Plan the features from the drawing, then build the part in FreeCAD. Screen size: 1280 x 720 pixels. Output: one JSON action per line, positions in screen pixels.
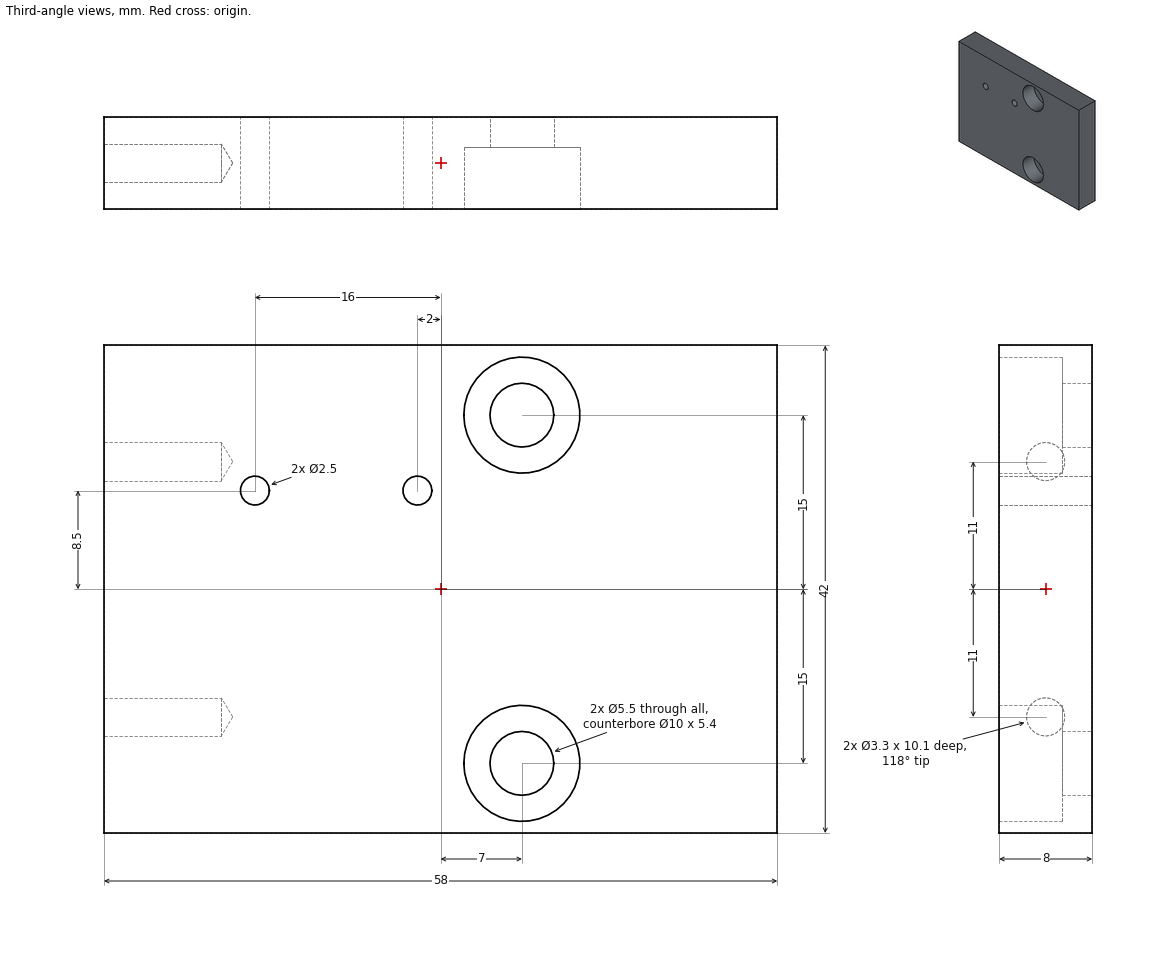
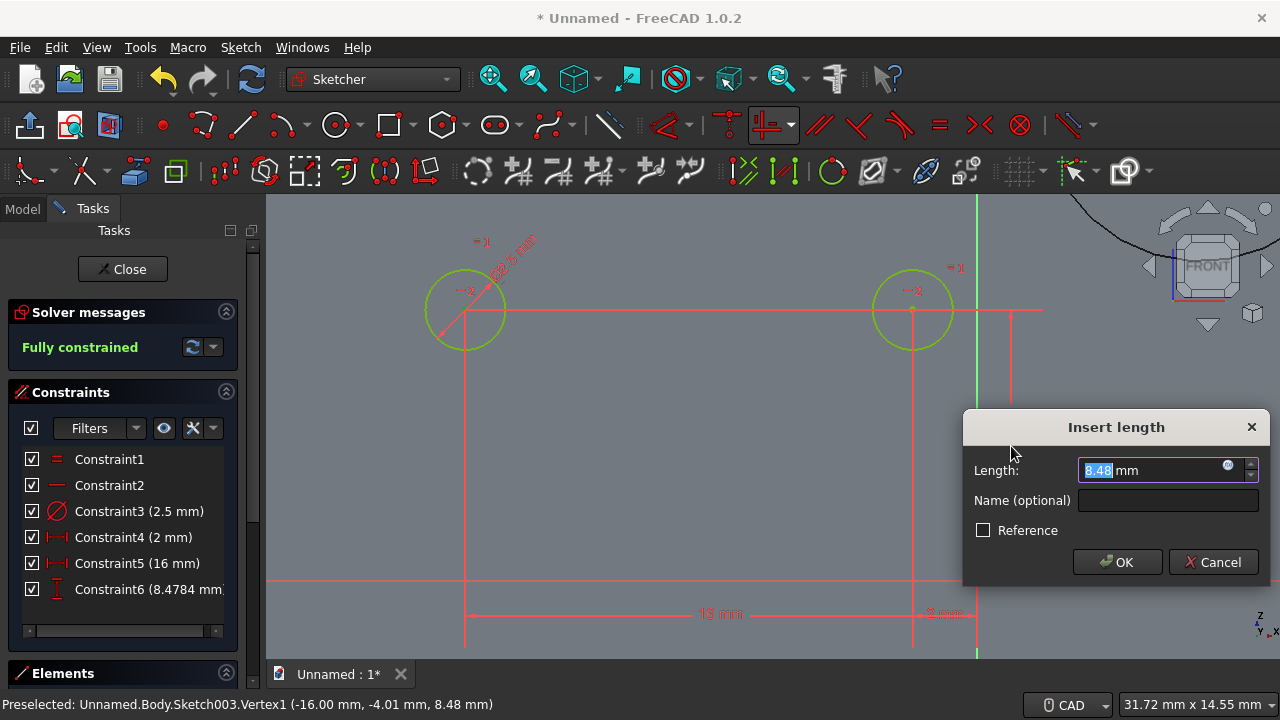
{"action": "type", "text": "8.5"}
{"action": "key", "text": "Return"}
{"action": "key", "text": "Escape"}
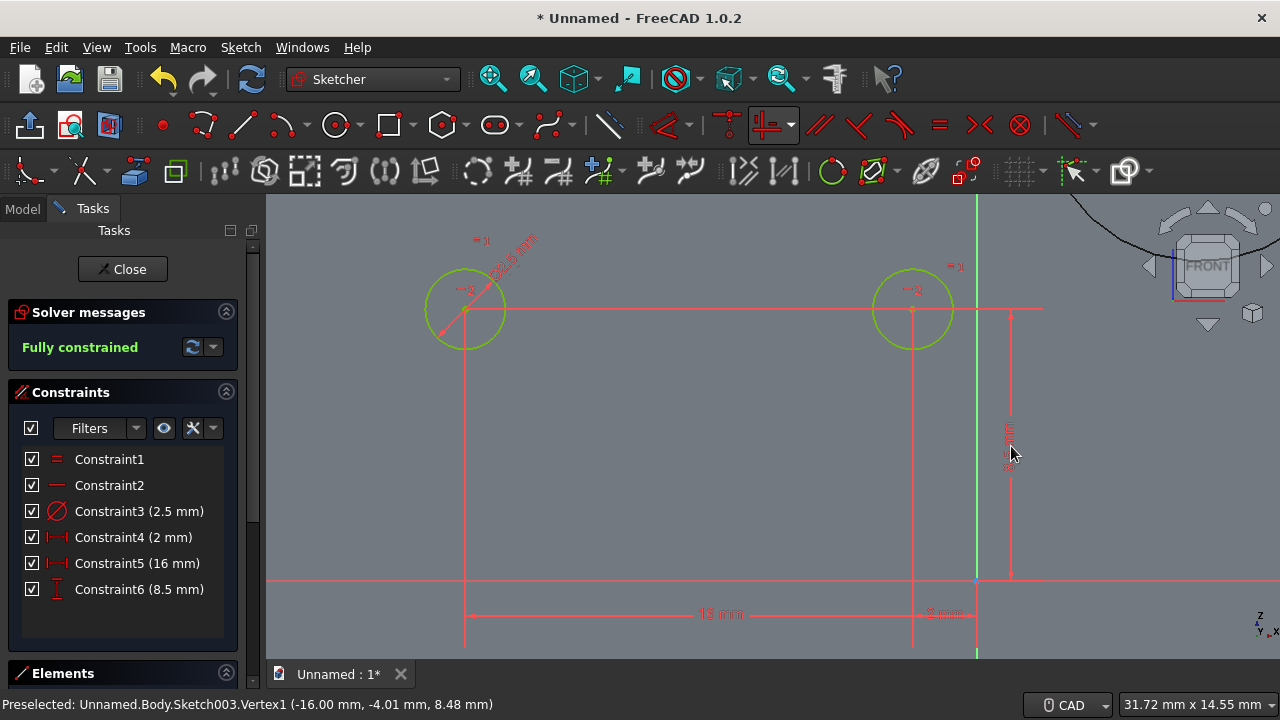
{"action": "left_click", "coordinate": [123, 269]}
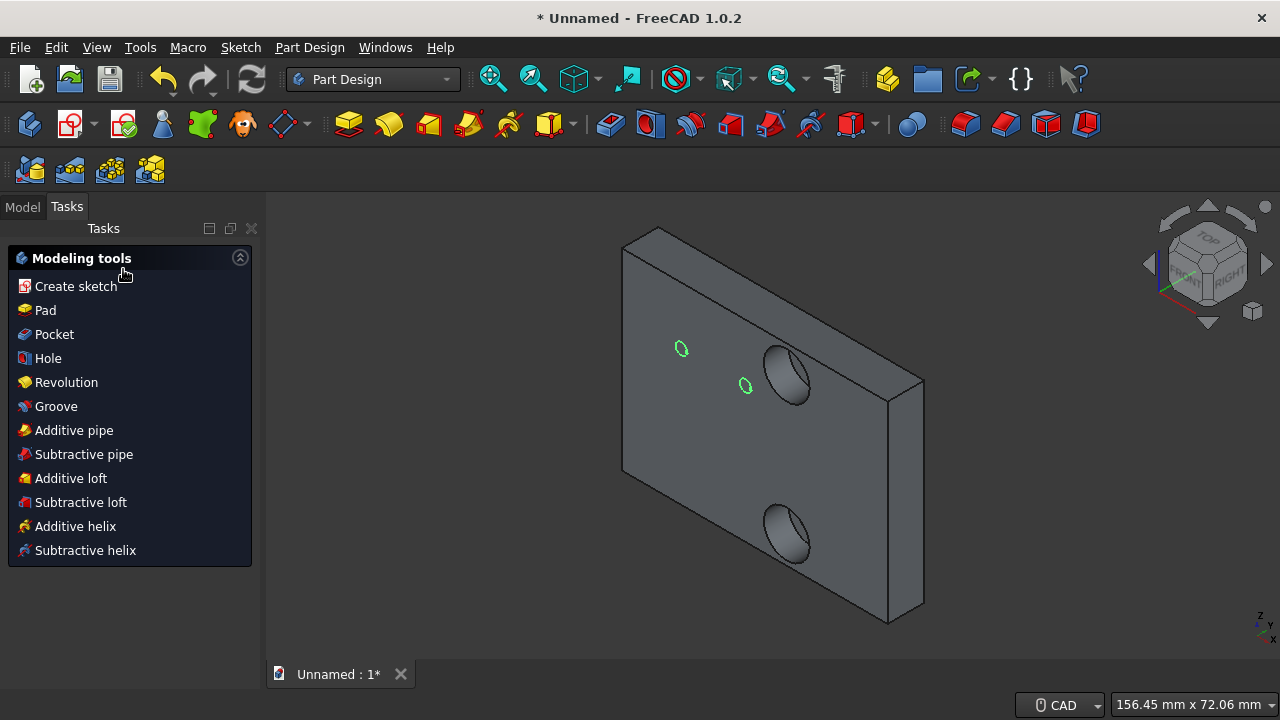
{"action": "left_click", "coordinate": [612, 124]}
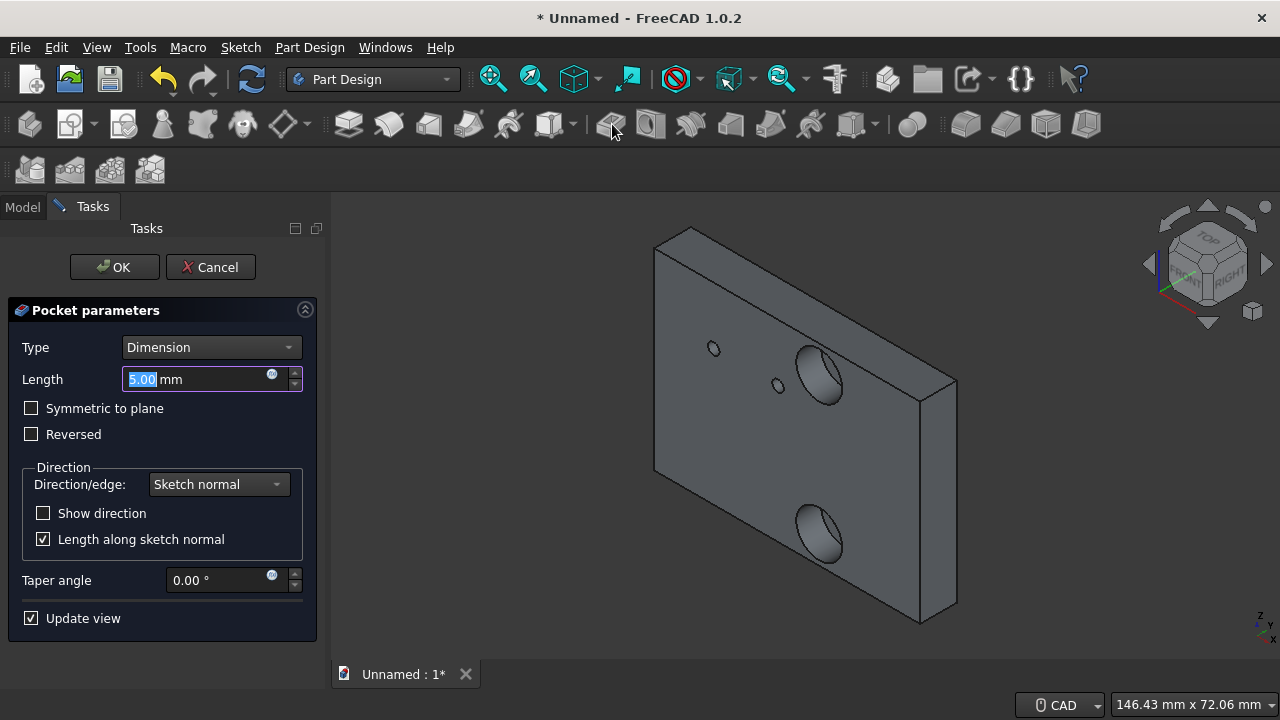
{"action": "left_click", "coordinate": [212, 348]}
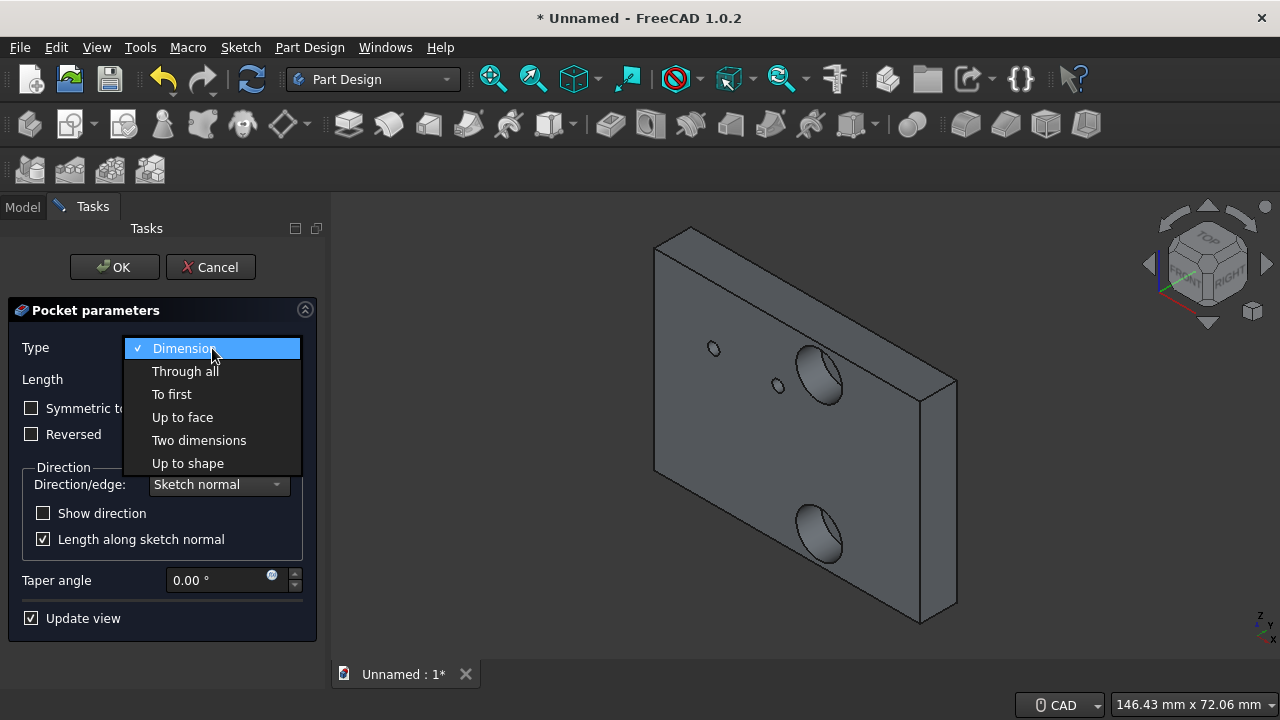
{"action": "left_click", "coordinate": [212, 372]}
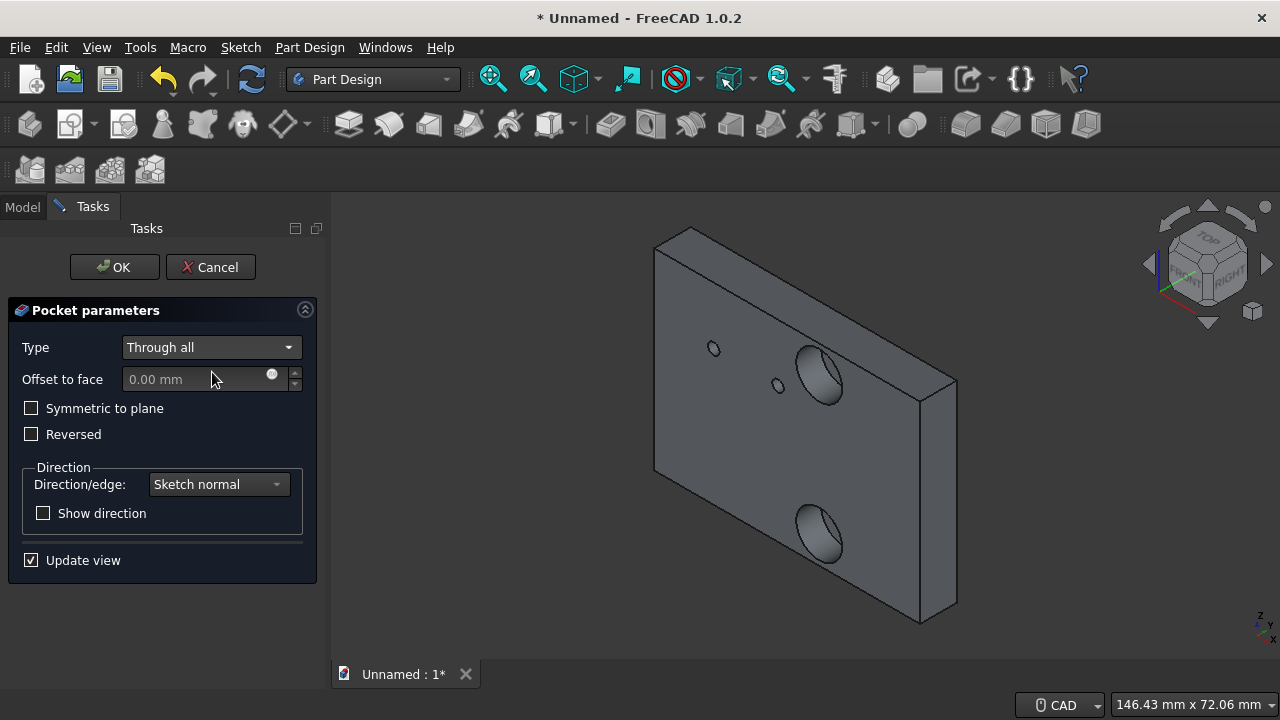
{"action": "left_click", "coordinate": [115, 267]}